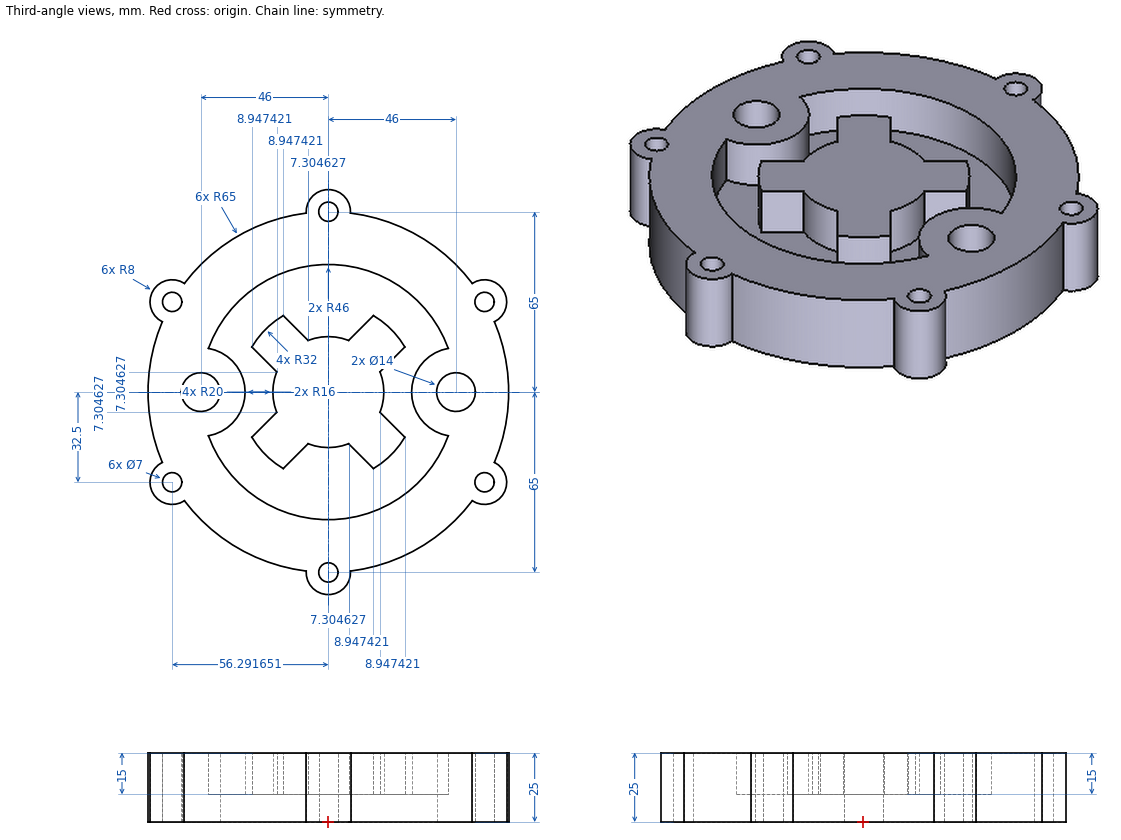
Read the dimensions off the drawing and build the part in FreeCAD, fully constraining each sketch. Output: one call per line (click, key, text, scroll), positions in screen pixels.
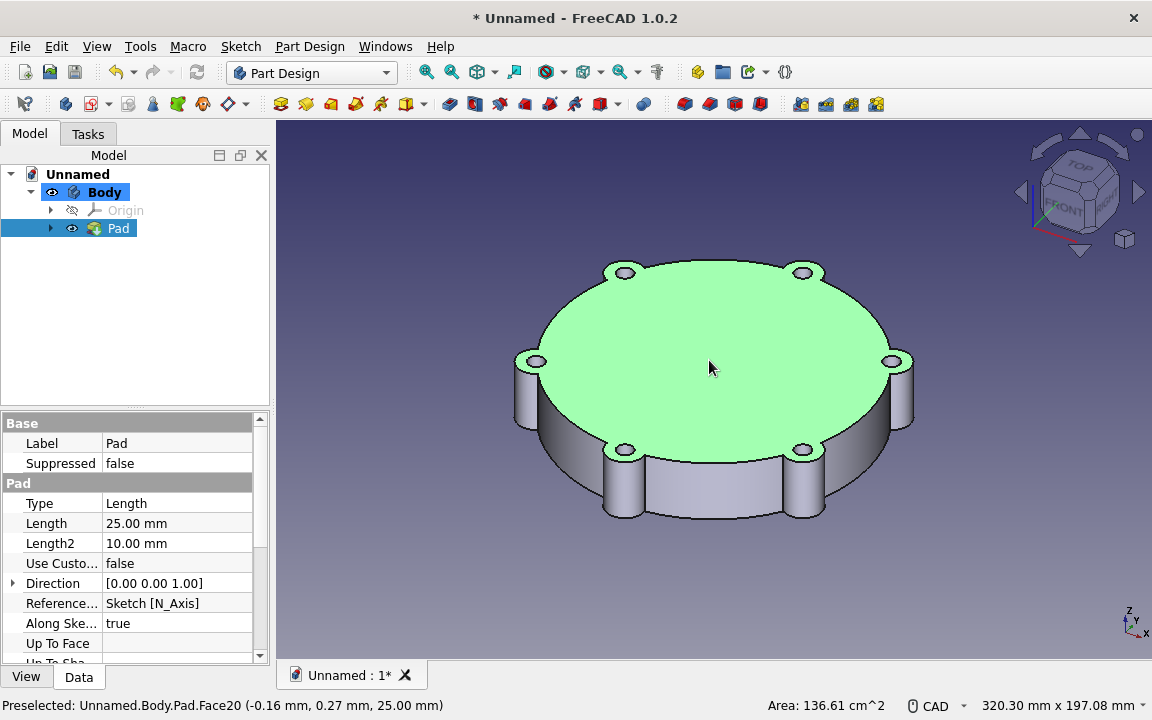
click(90, 104)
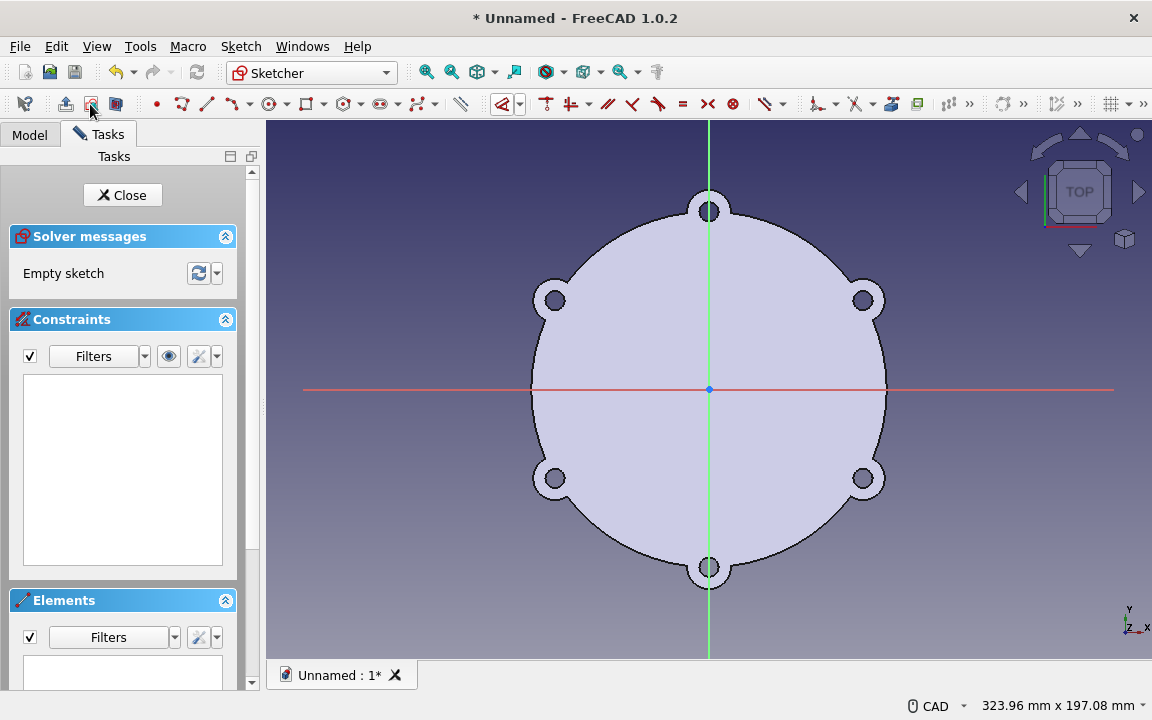
scroll(792, 389, up, 3)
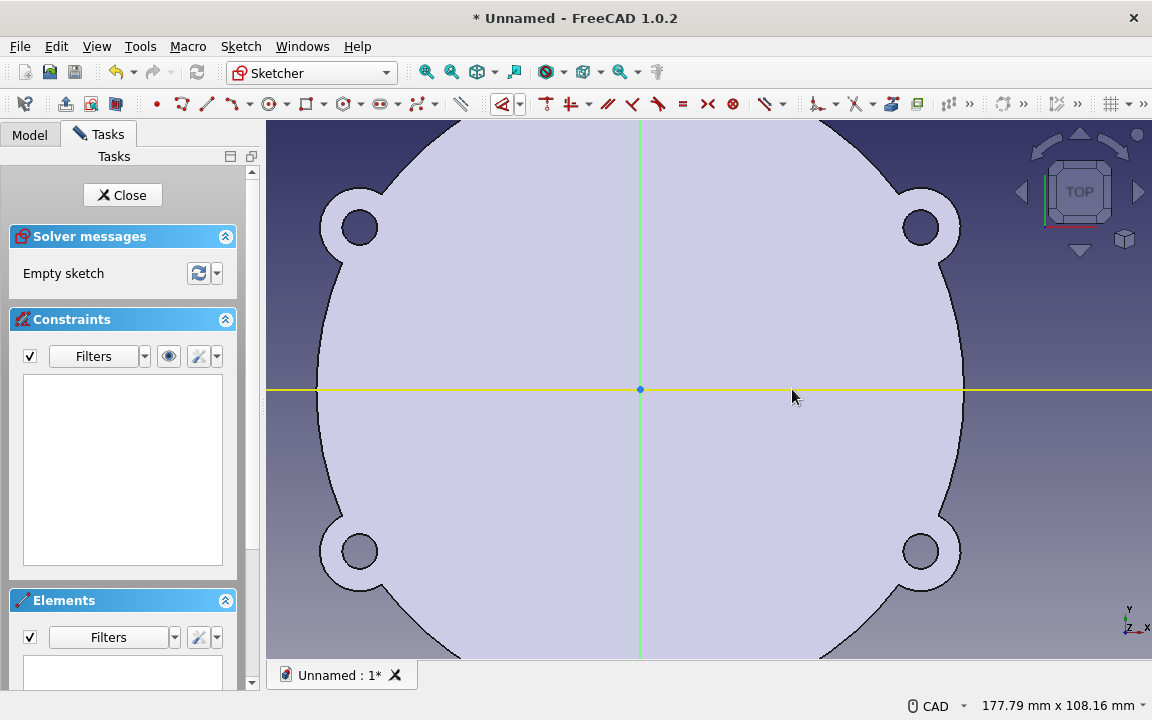
click(268, 104)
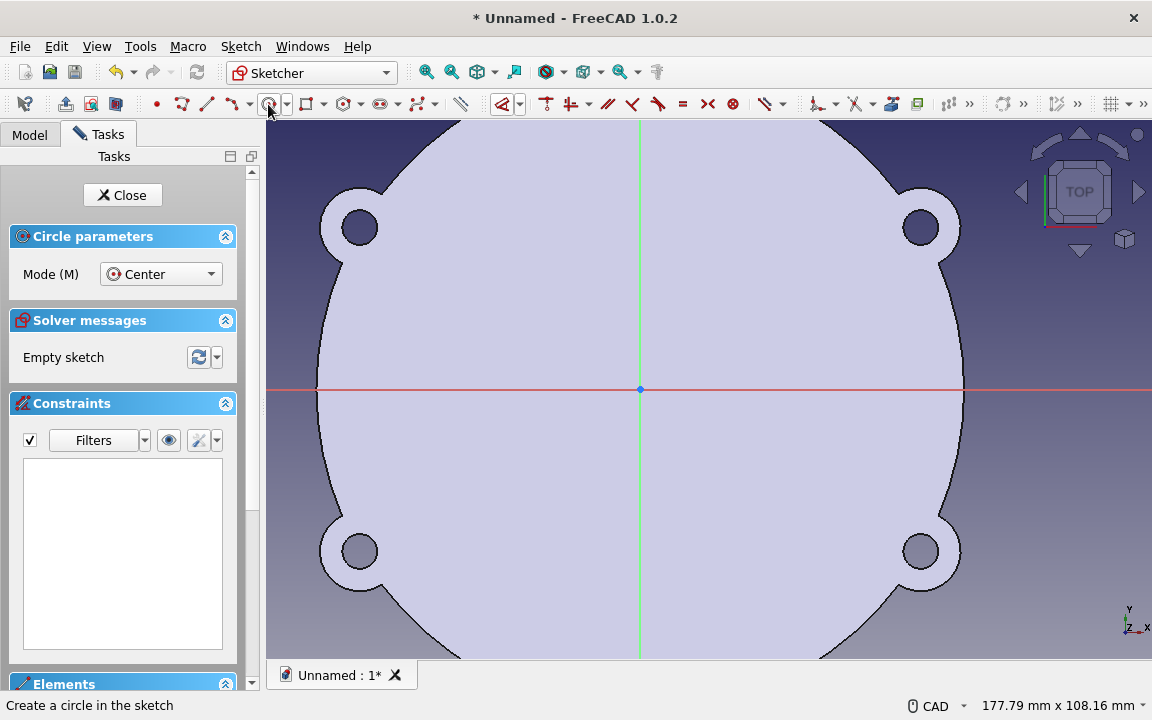
click(870, 390)
click(894, 365)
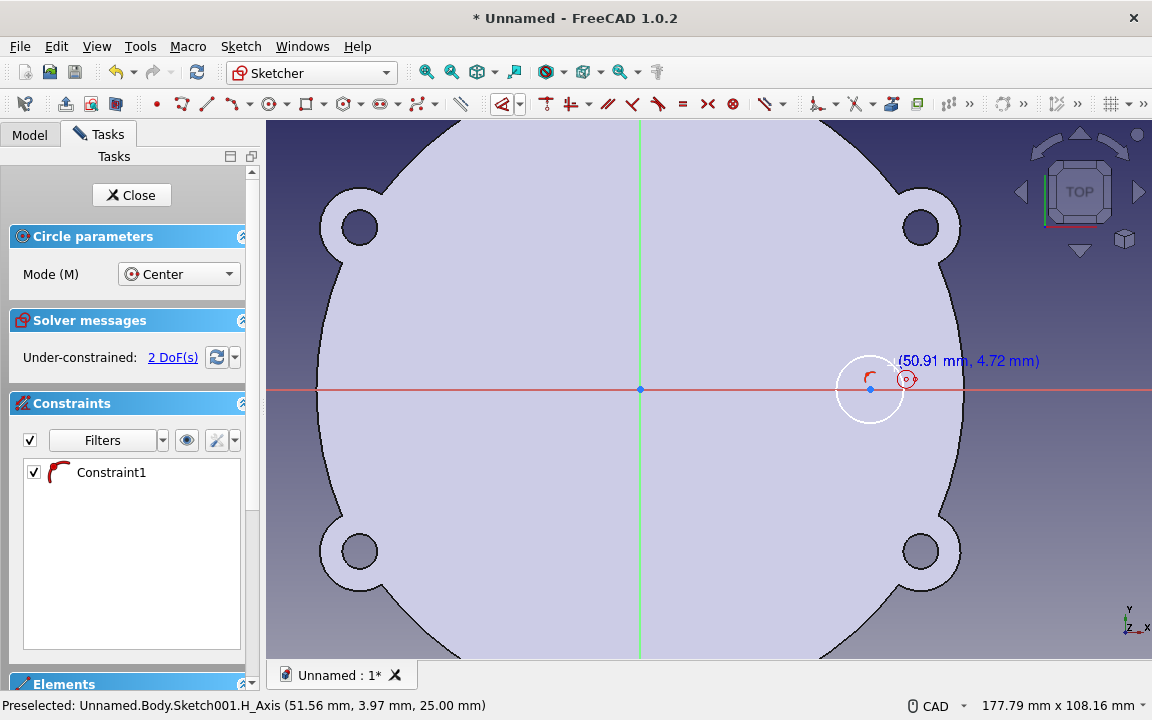
click(411, 390)
click(436, 365)
key(Escape)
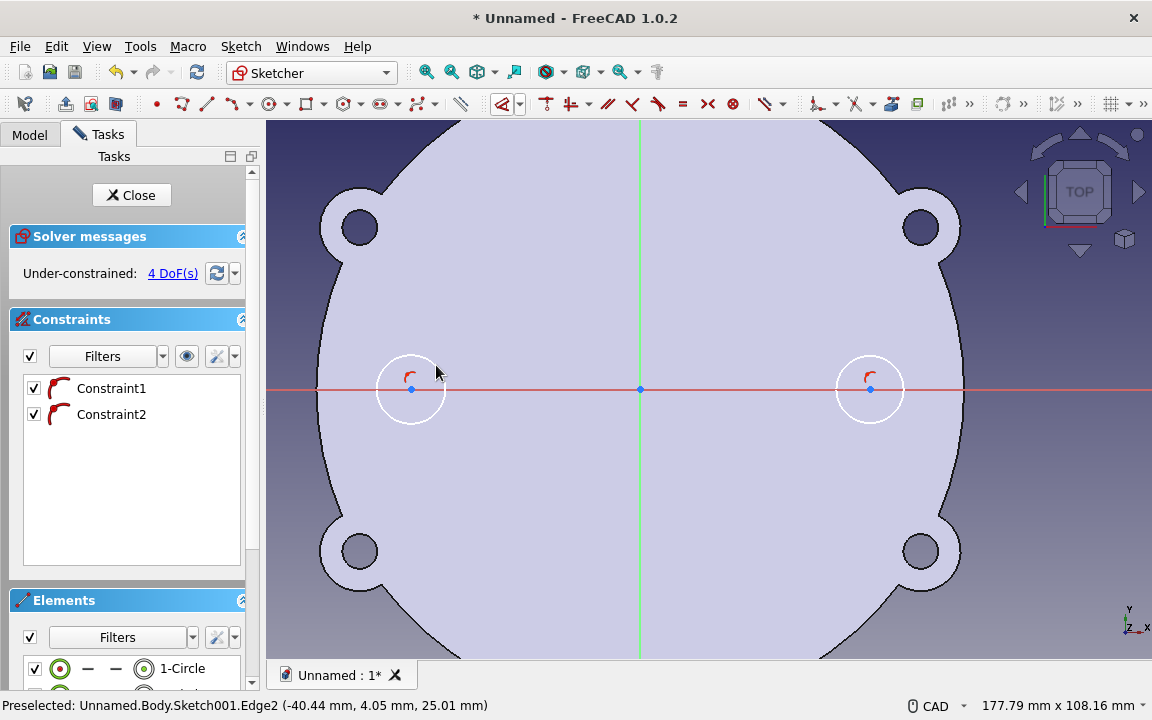
click(894, 366)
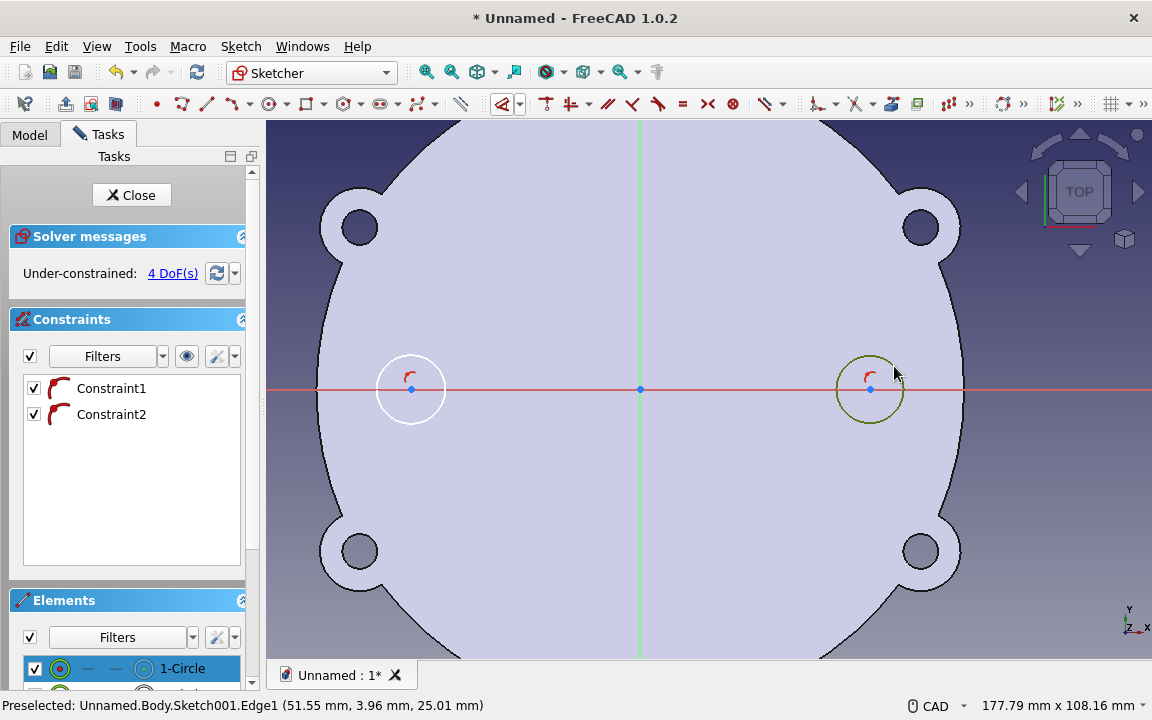
click(435, 365)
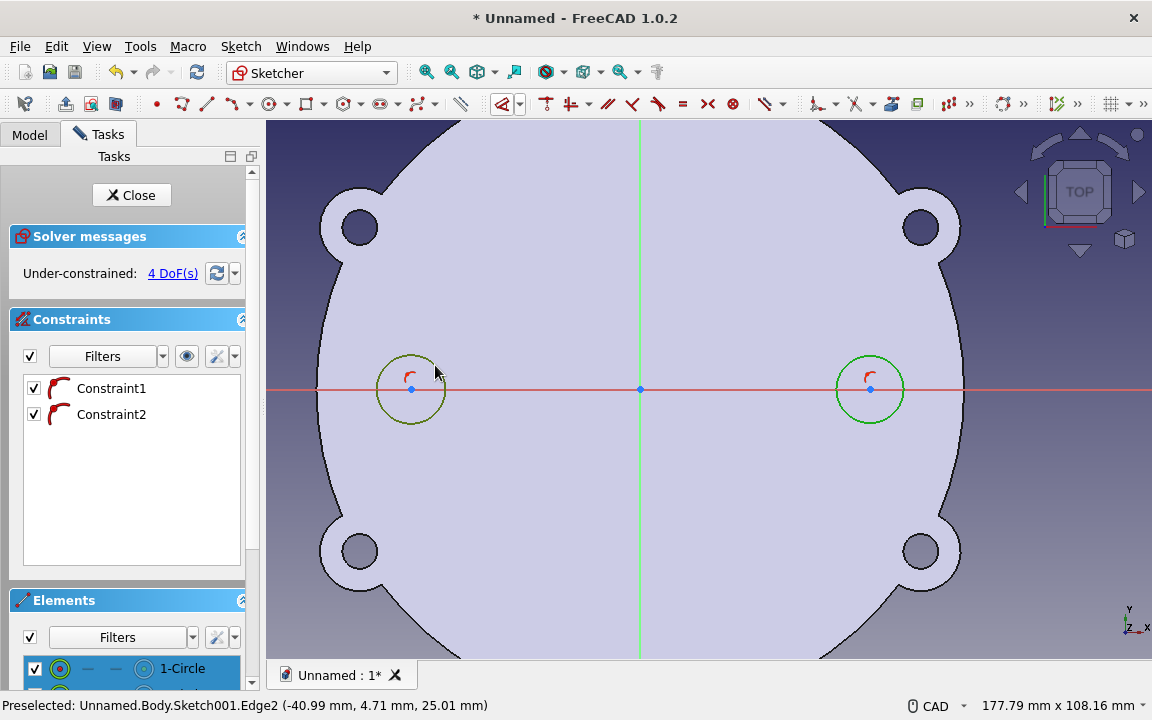
click(683, 104)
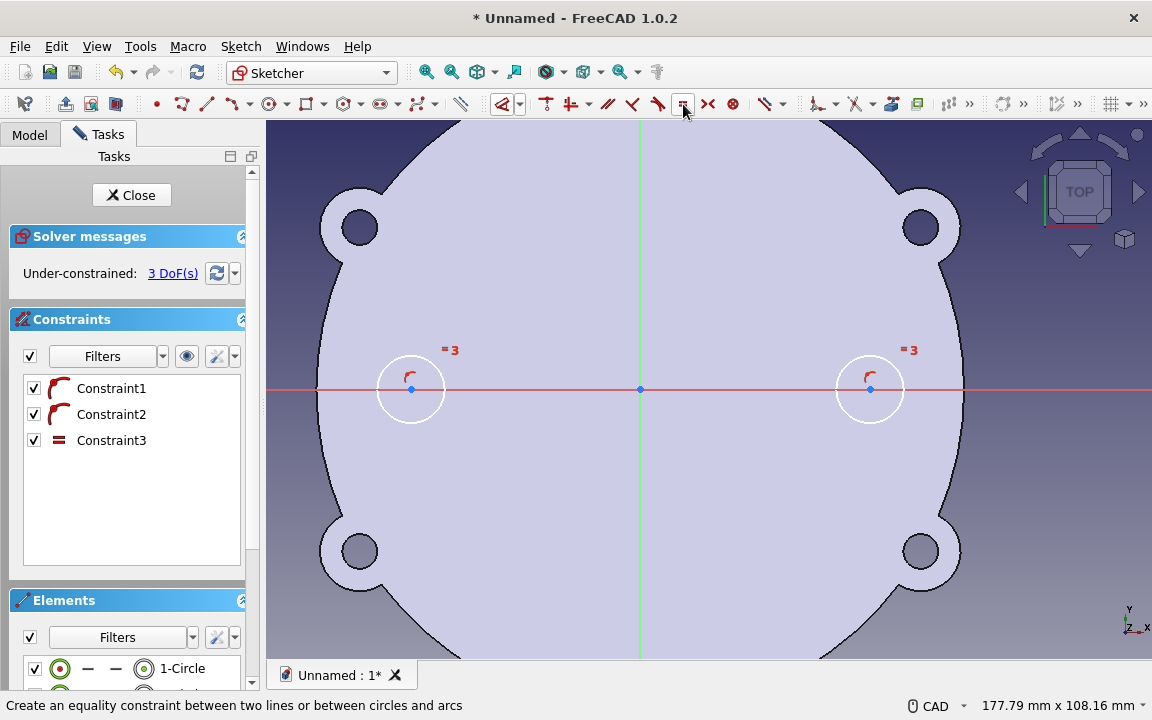
click(894, 366)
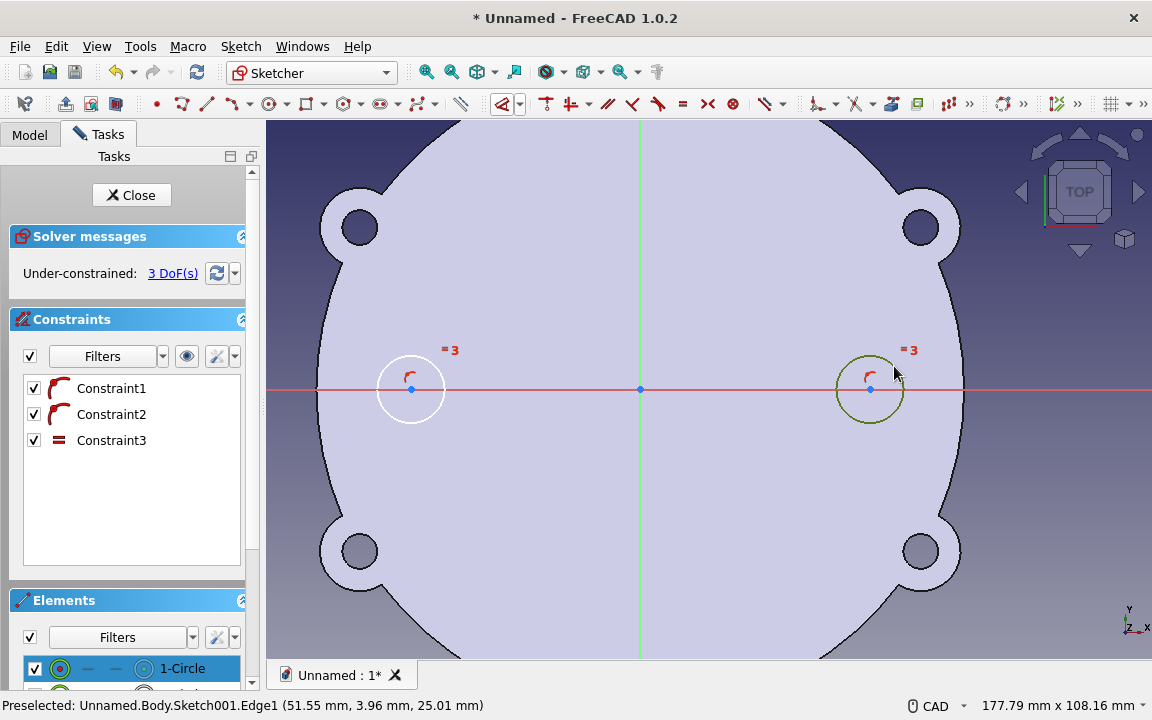
key(k)
key(o)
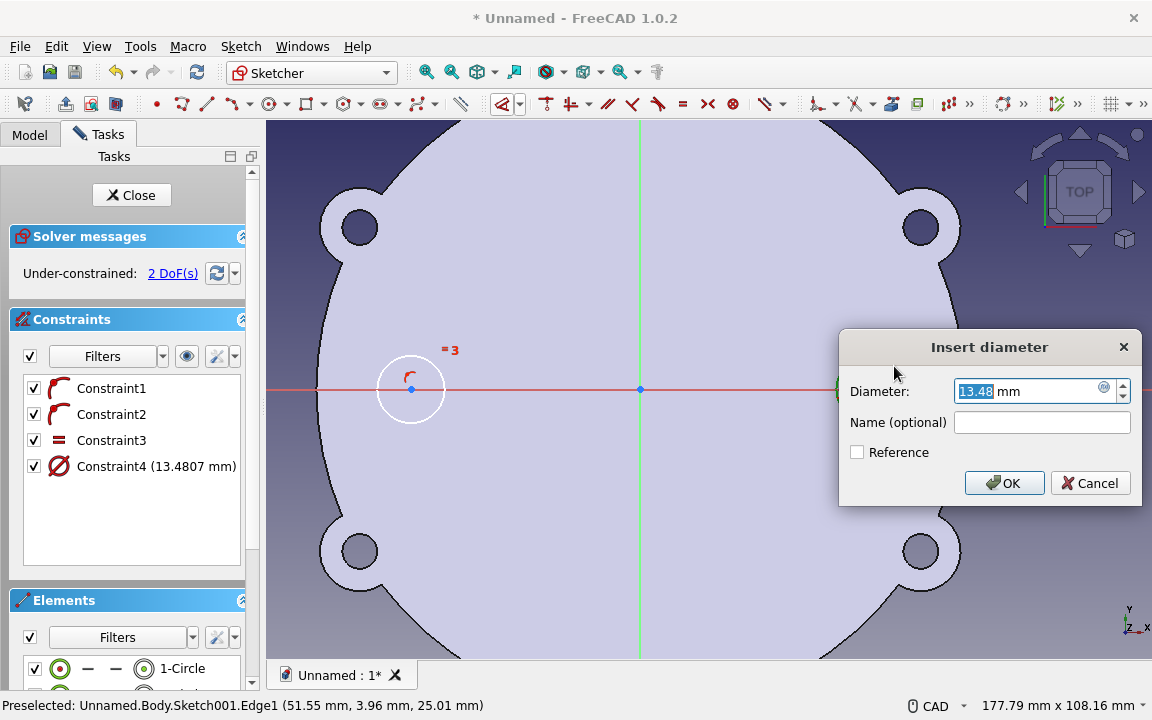
text(14)
key(Return)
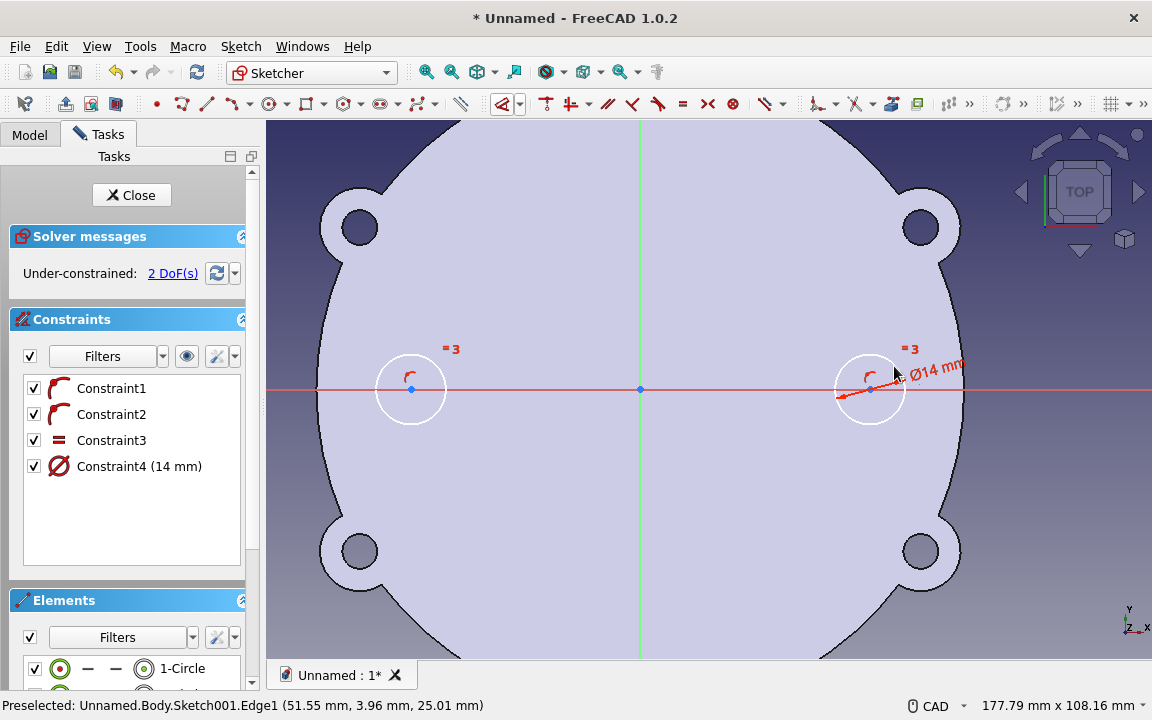
click(870, 390)